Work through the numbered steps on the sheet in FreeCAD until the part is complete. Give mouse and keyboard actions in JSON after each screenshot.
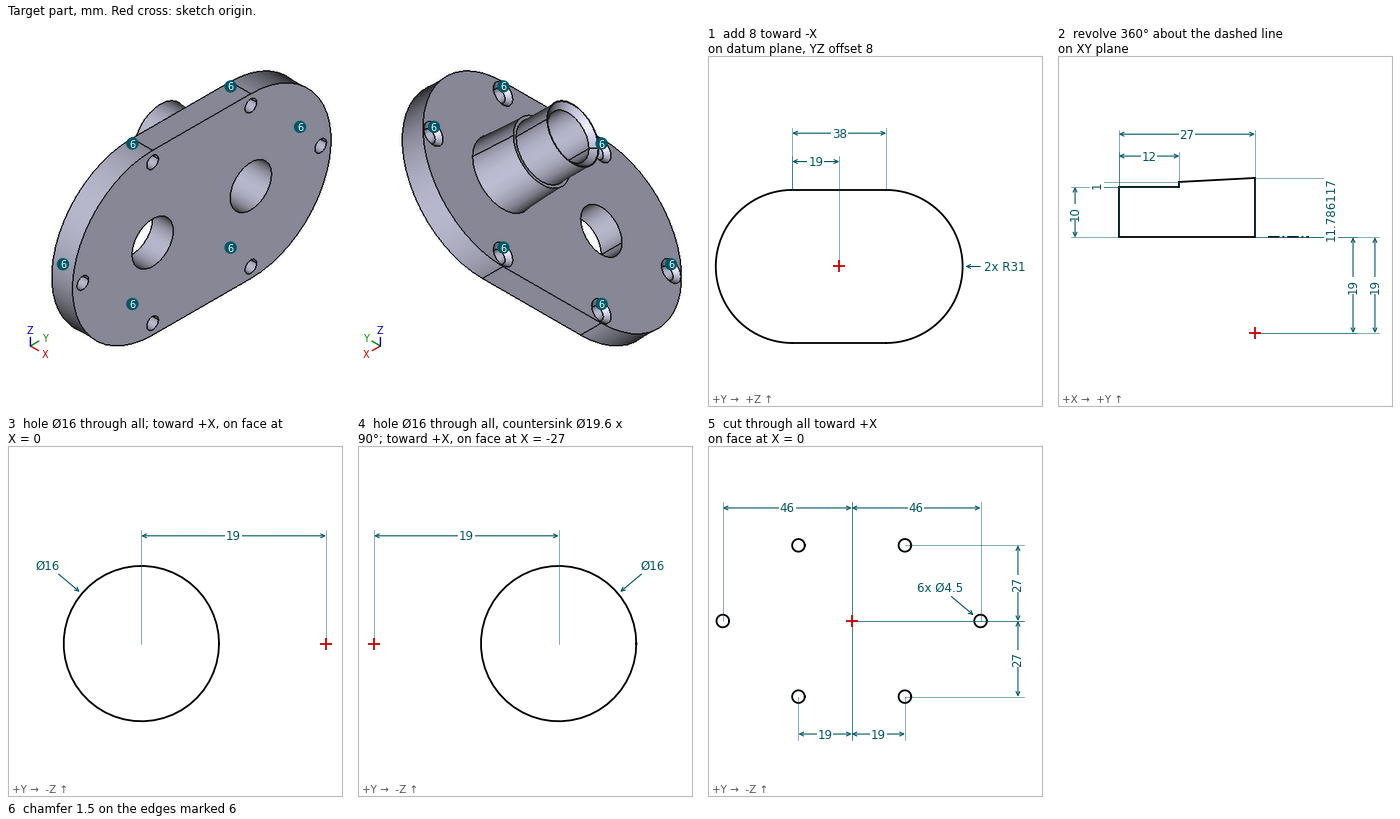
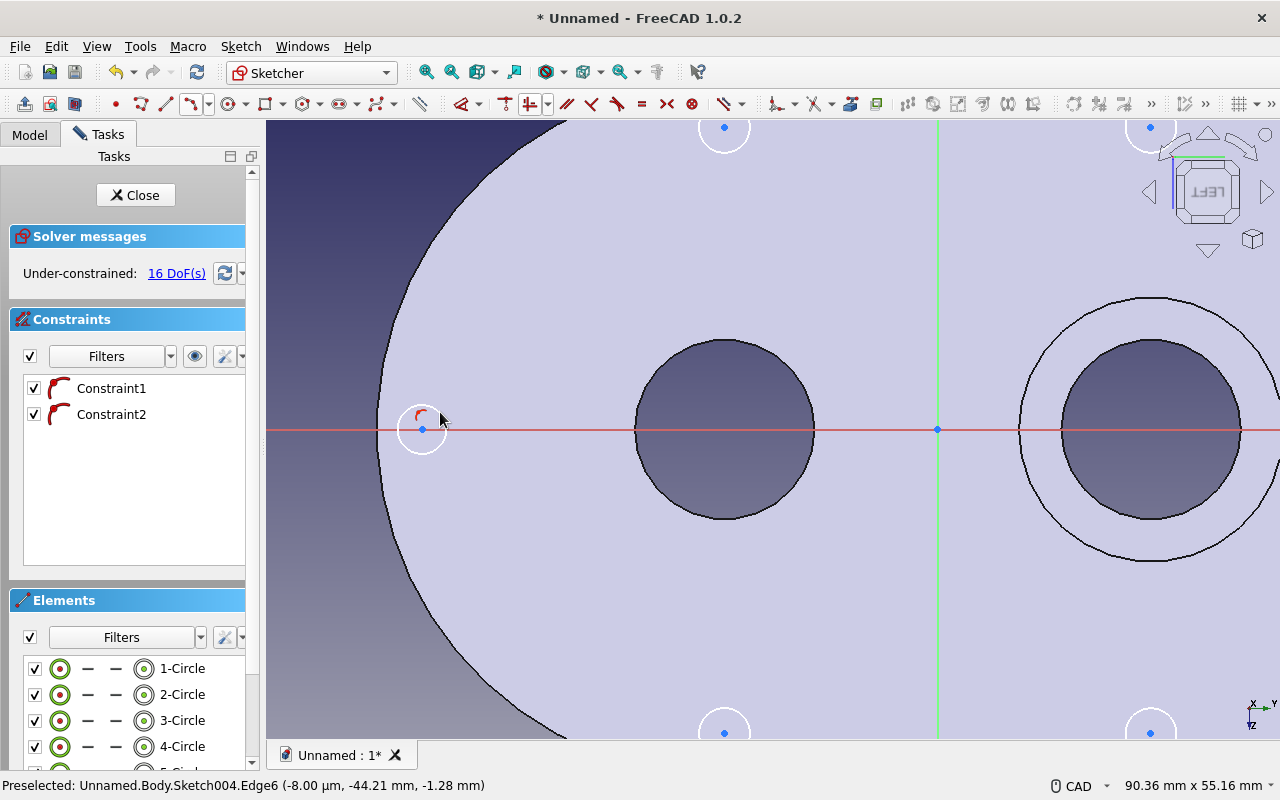
{"action": "scroll", "coordinate": [421, 430], "scroll_direction": "down", "scroll_amount": 3}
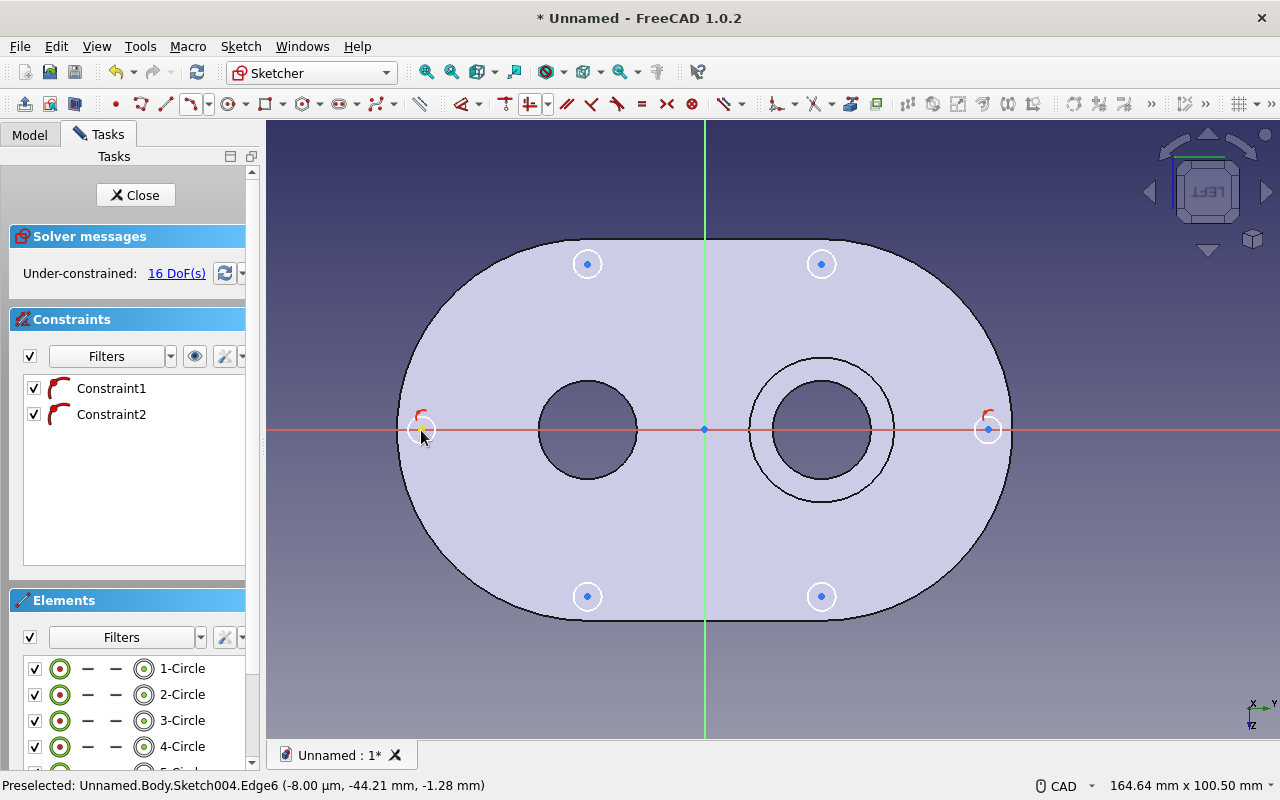
{"action": "scroll", "coordinate": [998, 420], "scroll_direction": "up", "scroll_amount": 2}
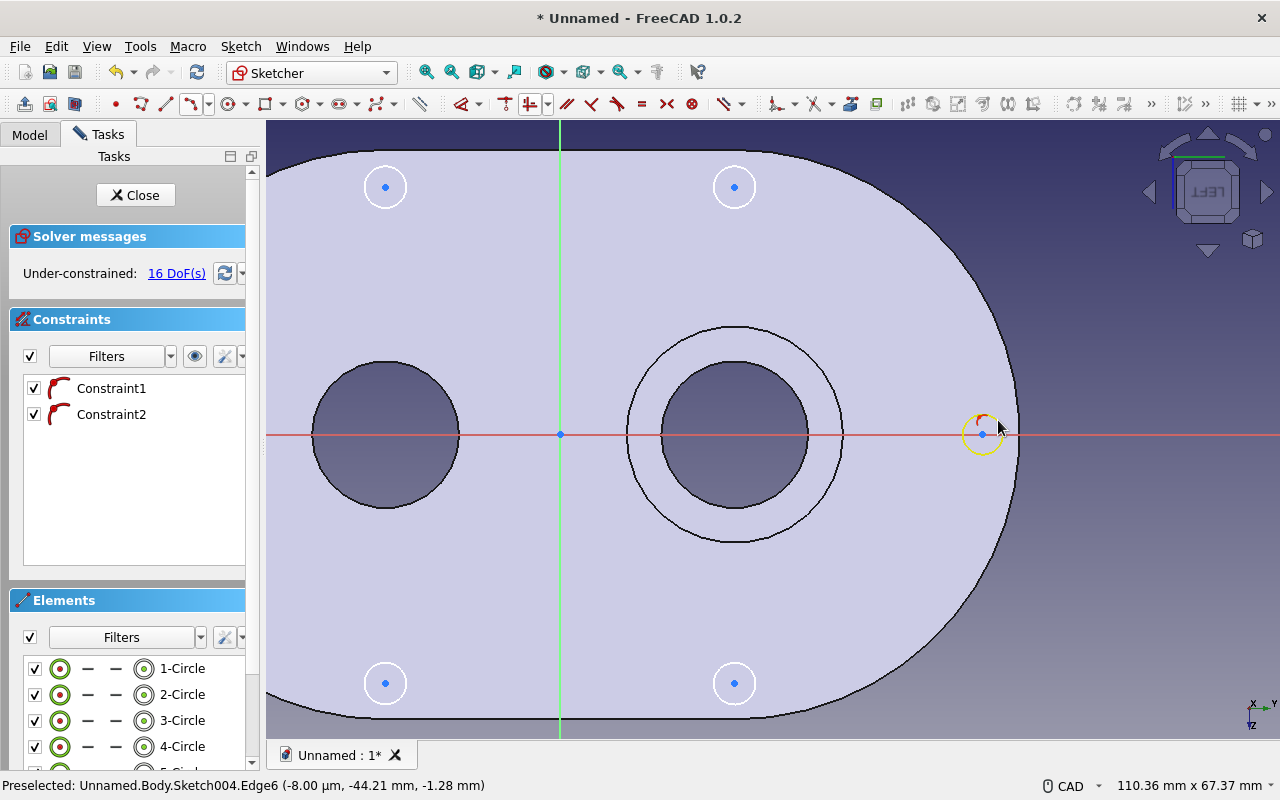
{"action": "left_click", "coordinate": [997, 420]}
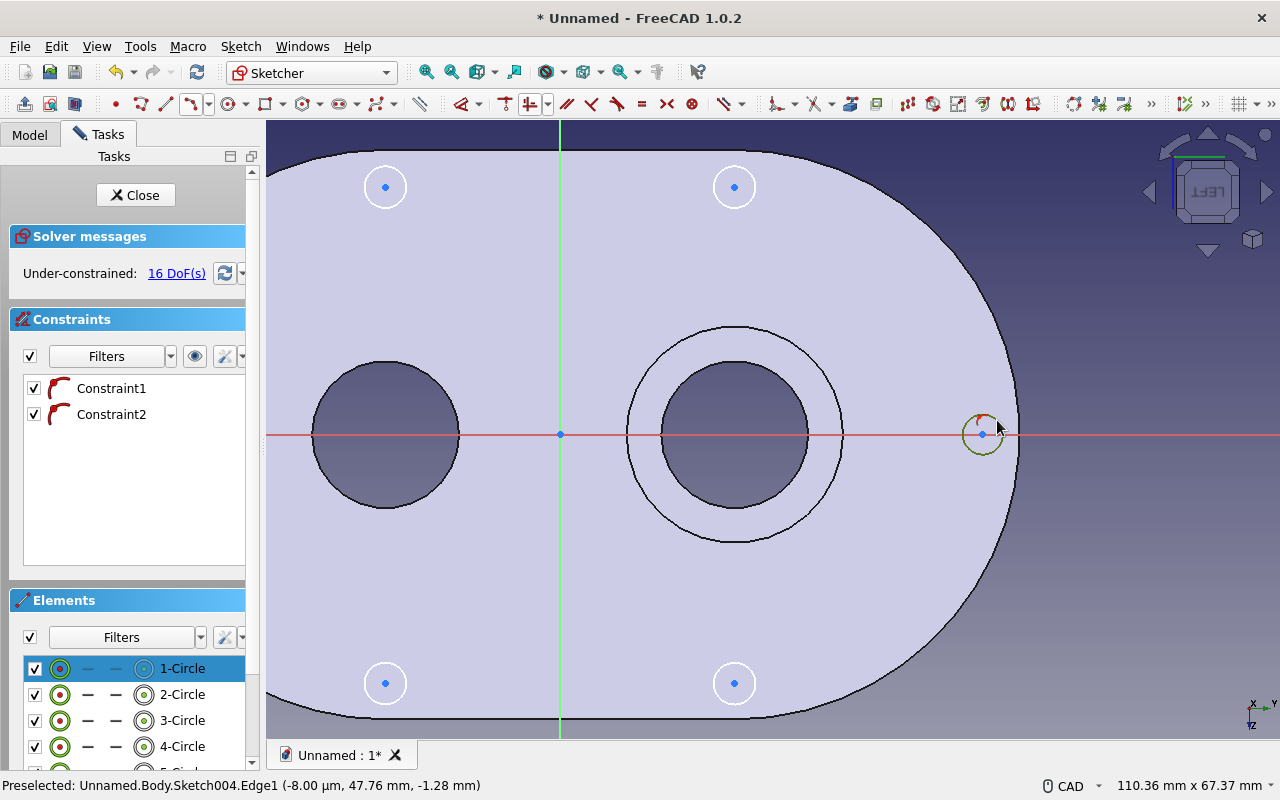
{"action": "left_click", "coordinate": [749, 669]}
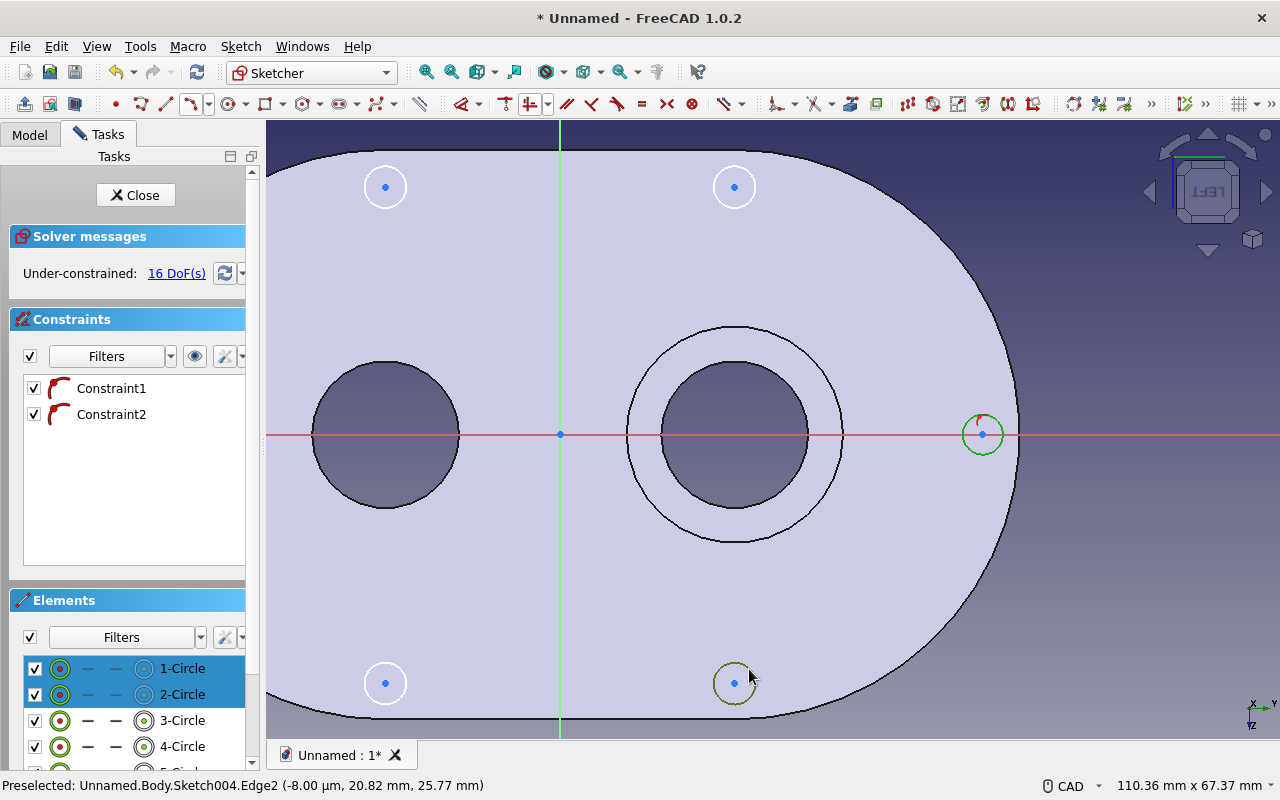
{"action": "left_click", "coordinate": [749, 172]}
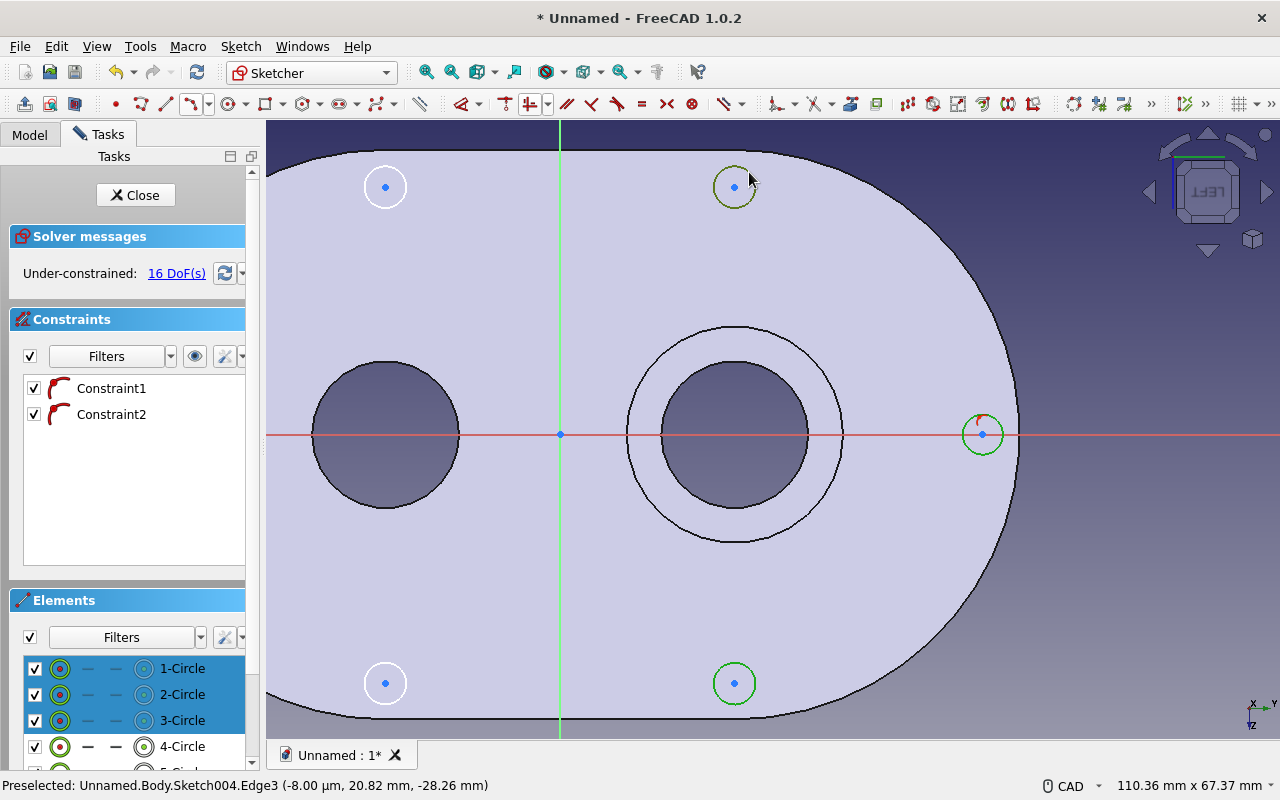
{"action": "left_click", "coordinate": [400, 669]}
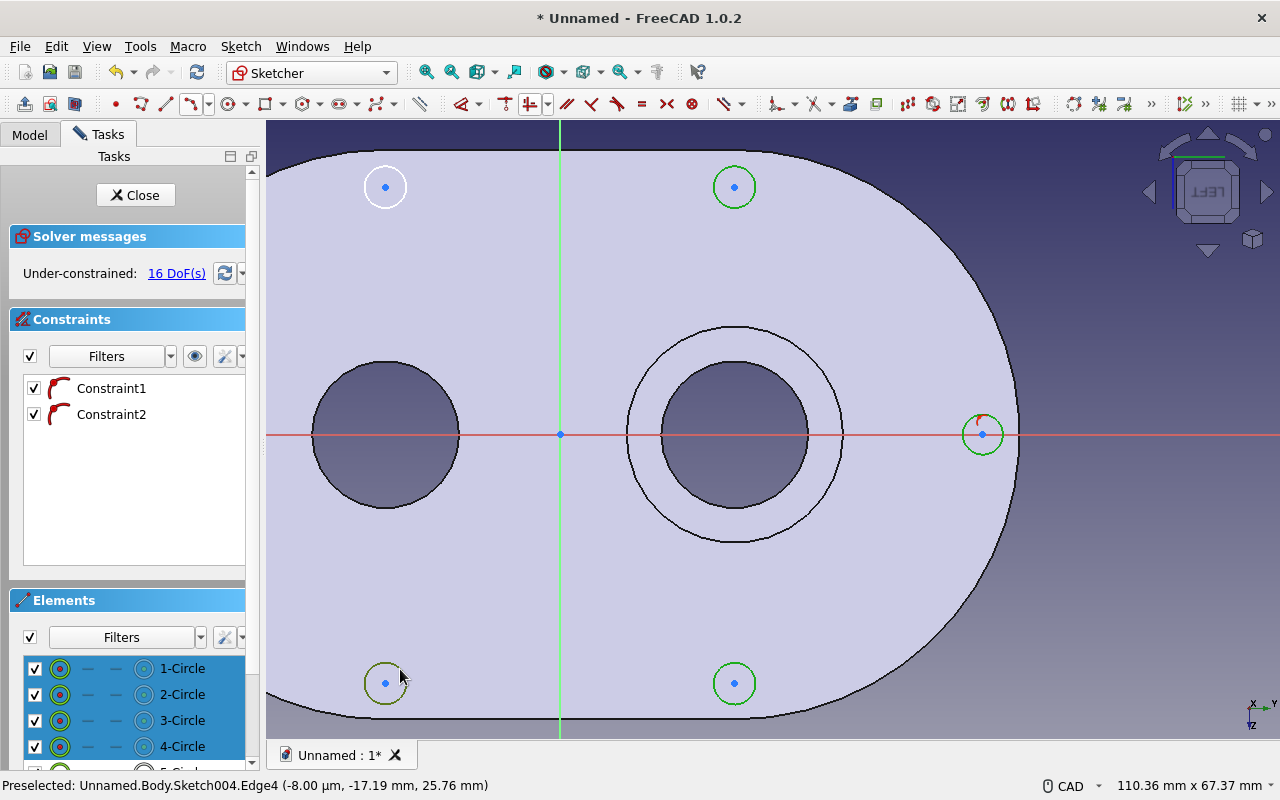
{"action": "left_click", "coordinate": [400, 172]}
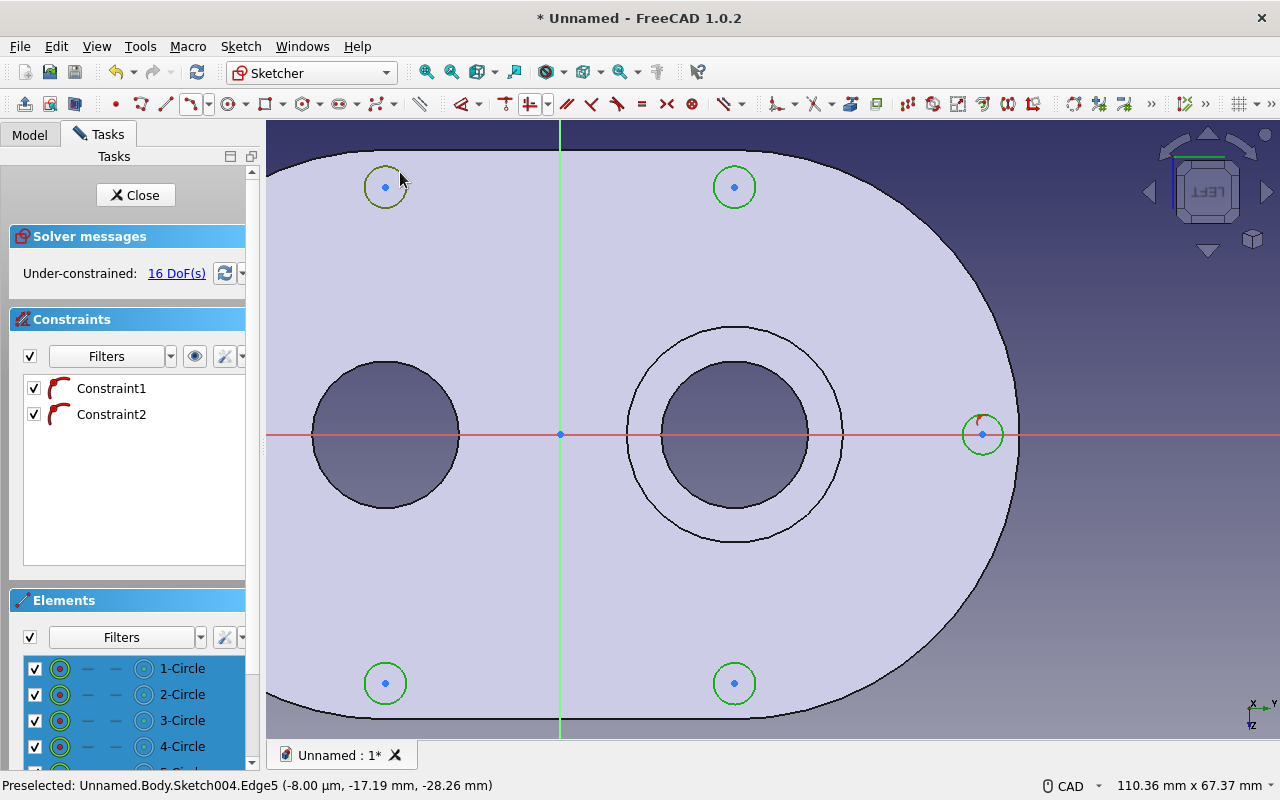
{"action": "scroll", "coordinate": [998, 419], "scroll_direction": "down", "scroll_amount": 2}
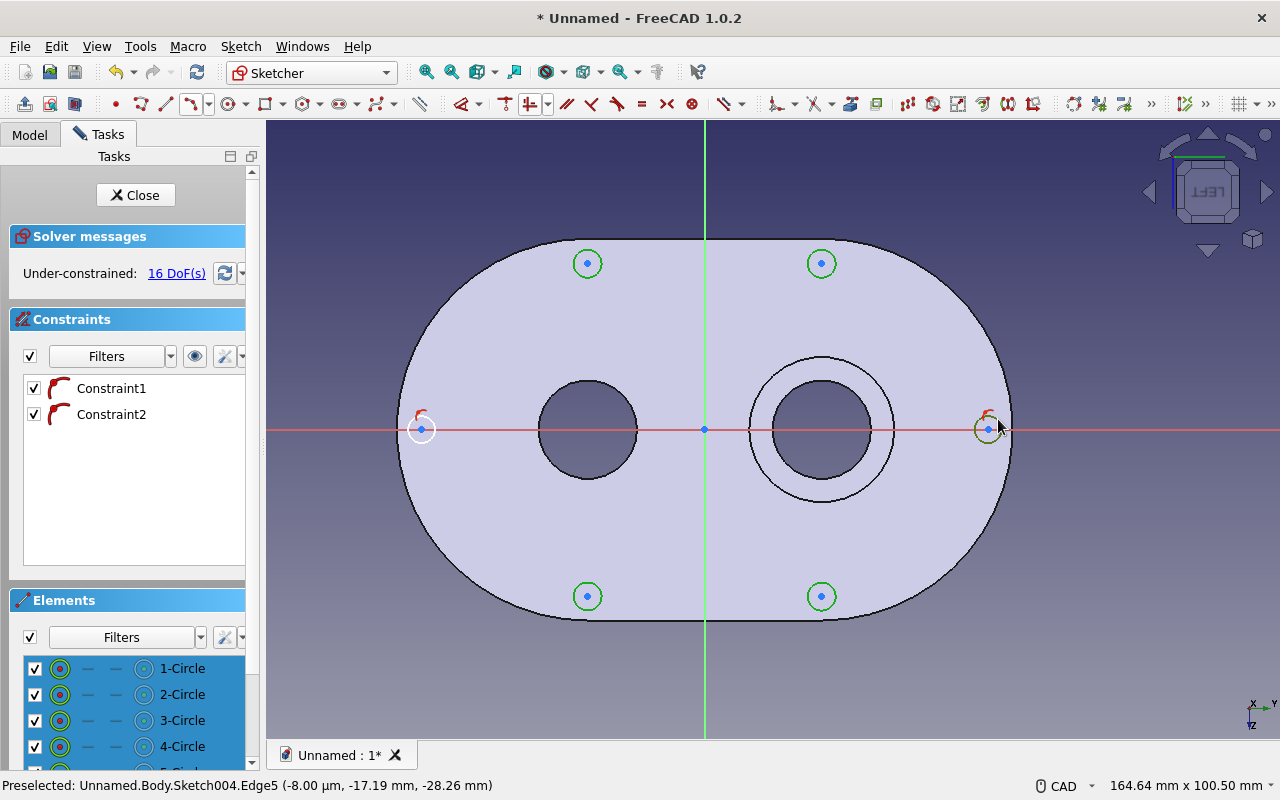
{"action": "scroll", "coordinate": [431, 420], "scroll_direction": "up", "scroll_amount": 2}